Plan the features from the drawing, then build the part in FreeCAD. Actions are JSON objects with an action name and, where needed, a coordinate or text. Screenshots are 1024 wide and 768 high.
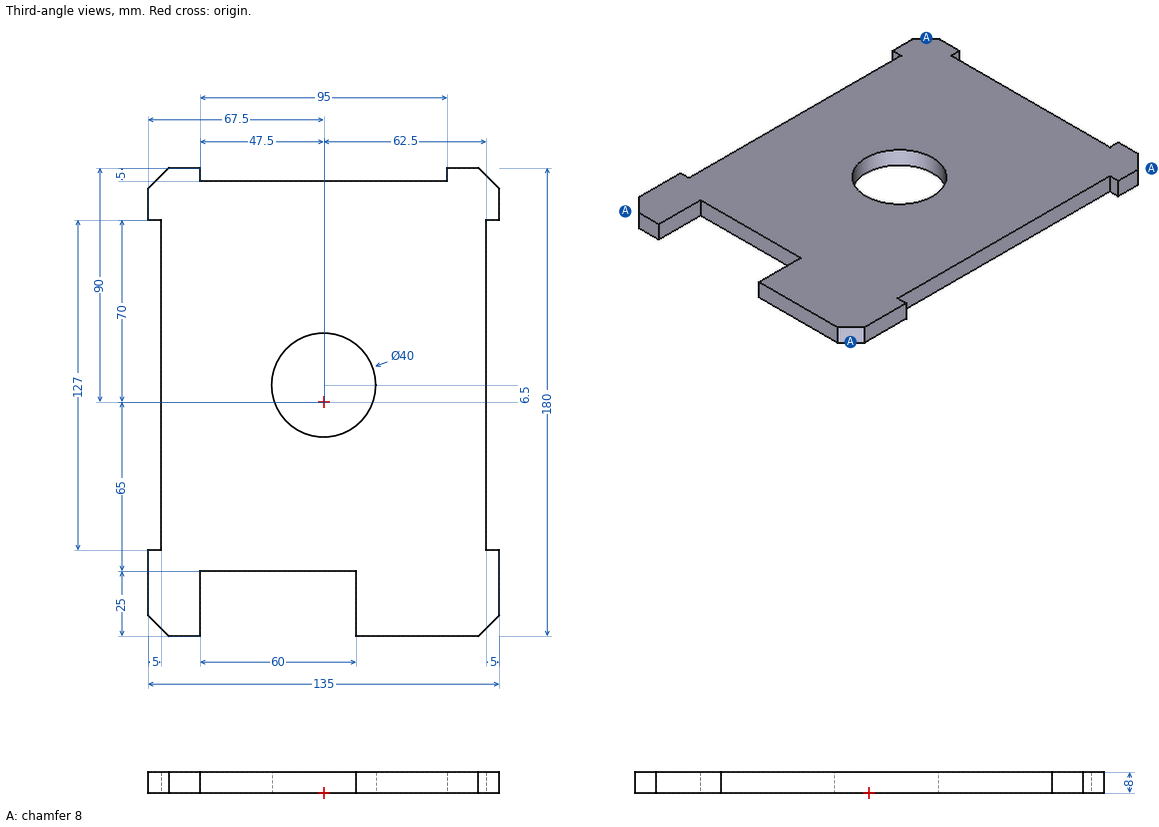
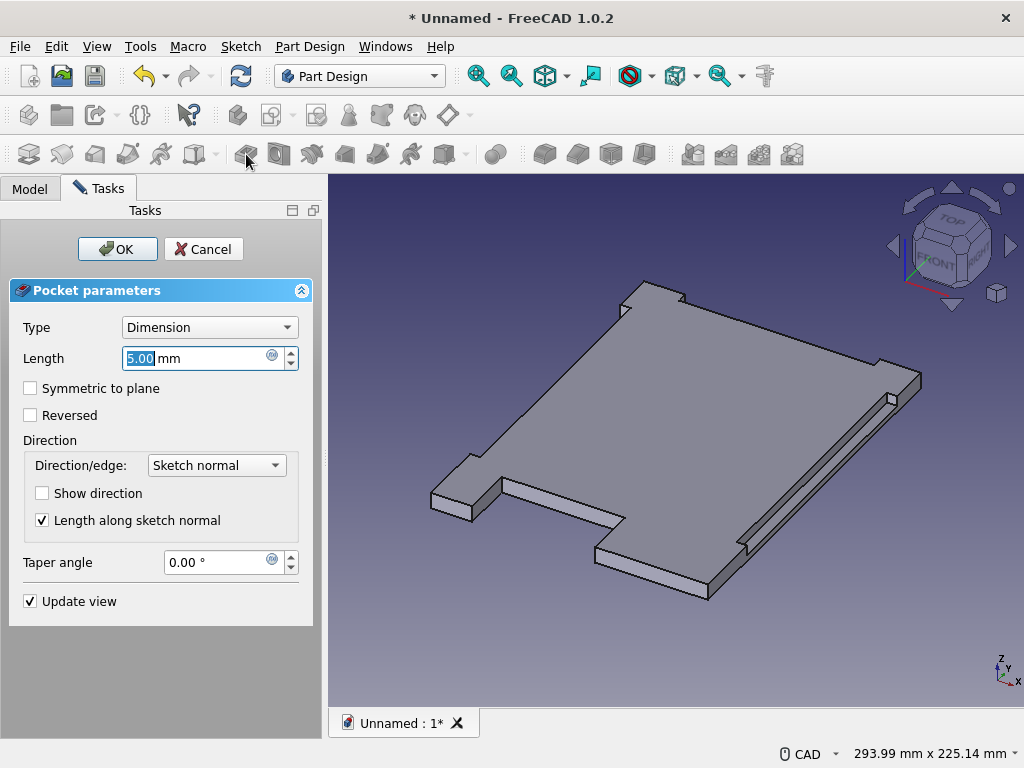
{"action": "left_click", "coordinate": [210, 328]}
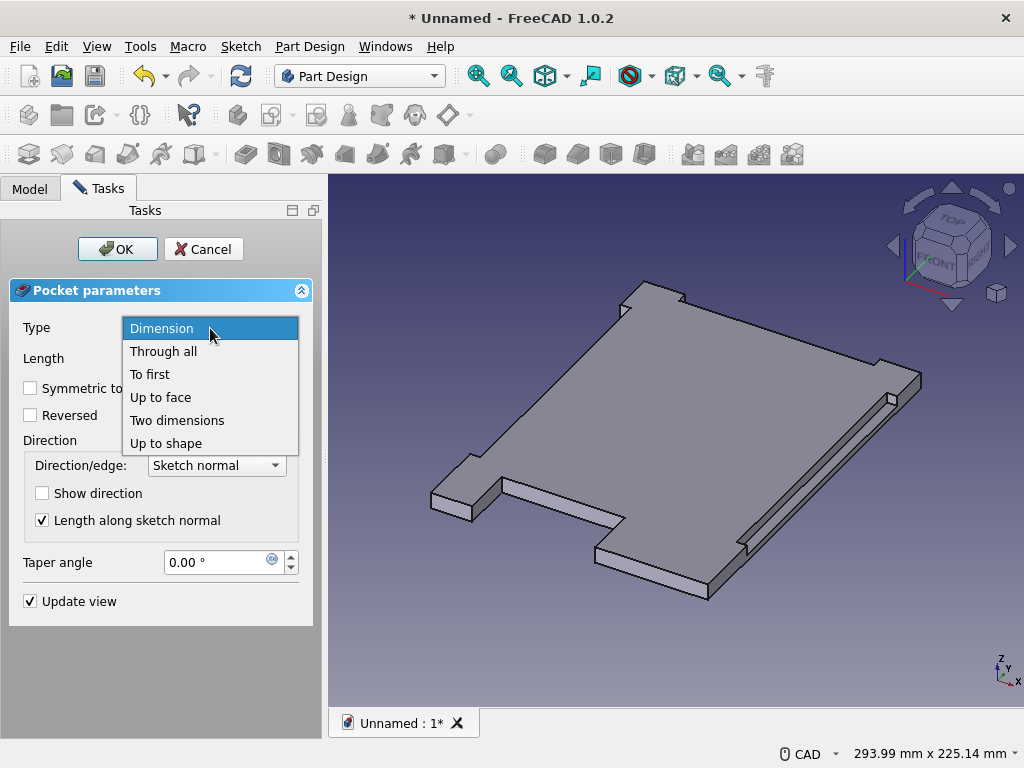
{"action": "left_click", "coordinate": [208, 374]}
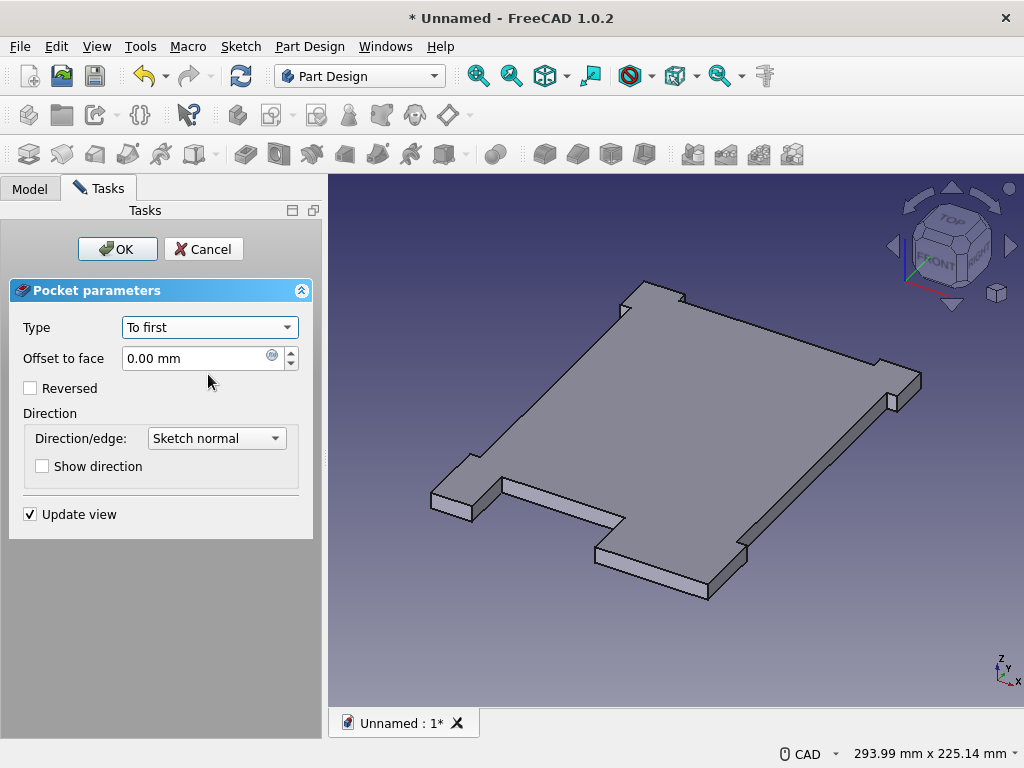
{"action": "left_click", "coordinate": [118, 249]}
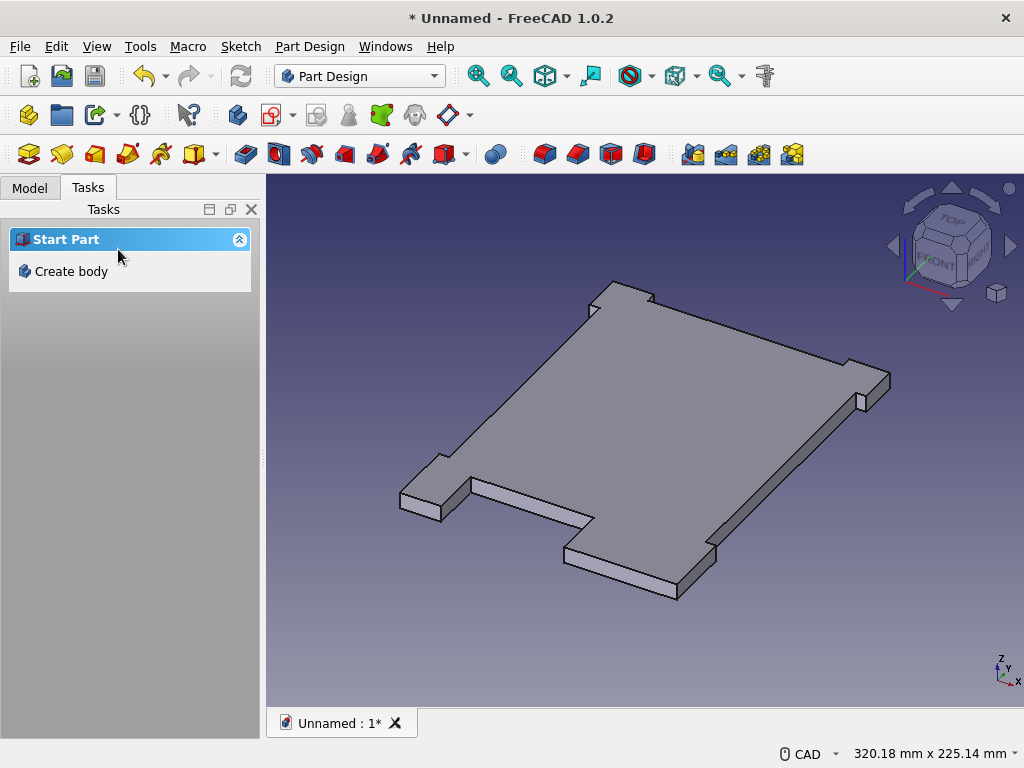
{"action": "left_click", "coordinate": [677, 591]}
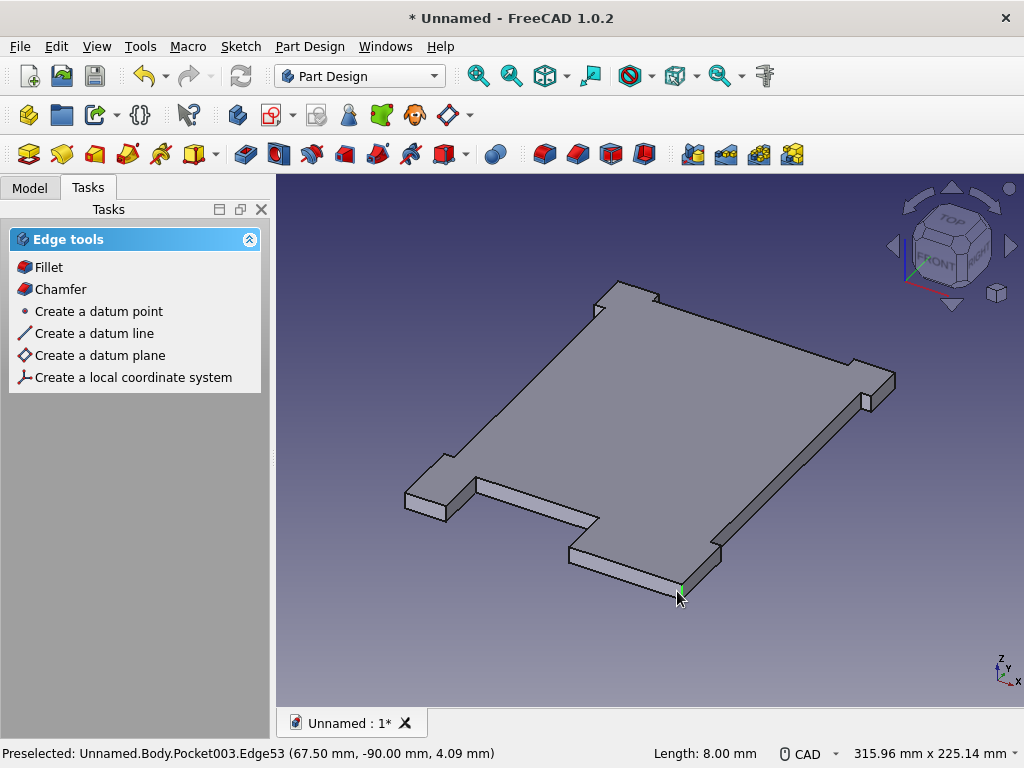
{"action": "scroll", "coordinate": [405, 500], "scroll_direction": "up", "scroll_amount": 4}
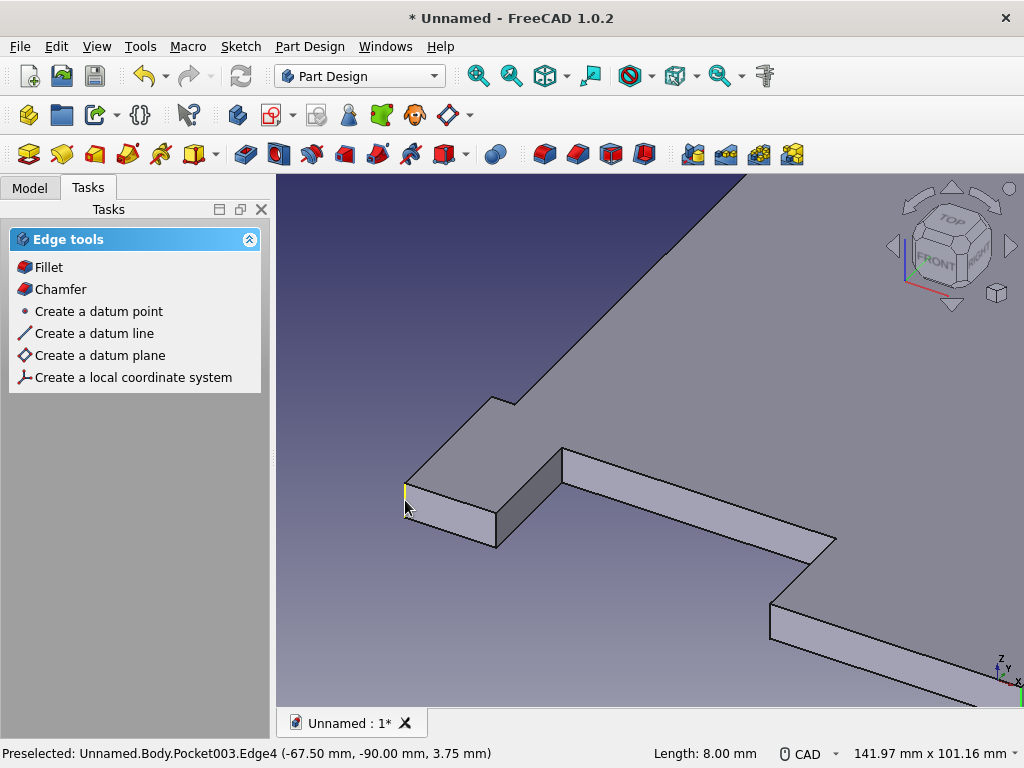
{"action": "key", "text": "v f"}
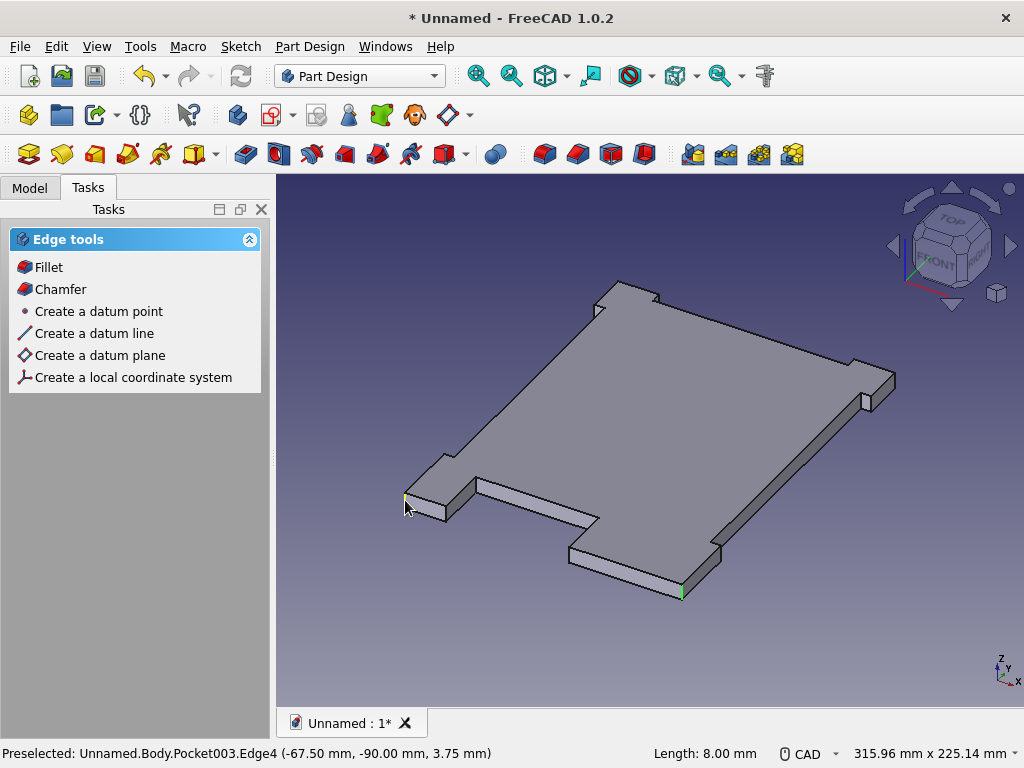
{"action": "key", "text": "0"}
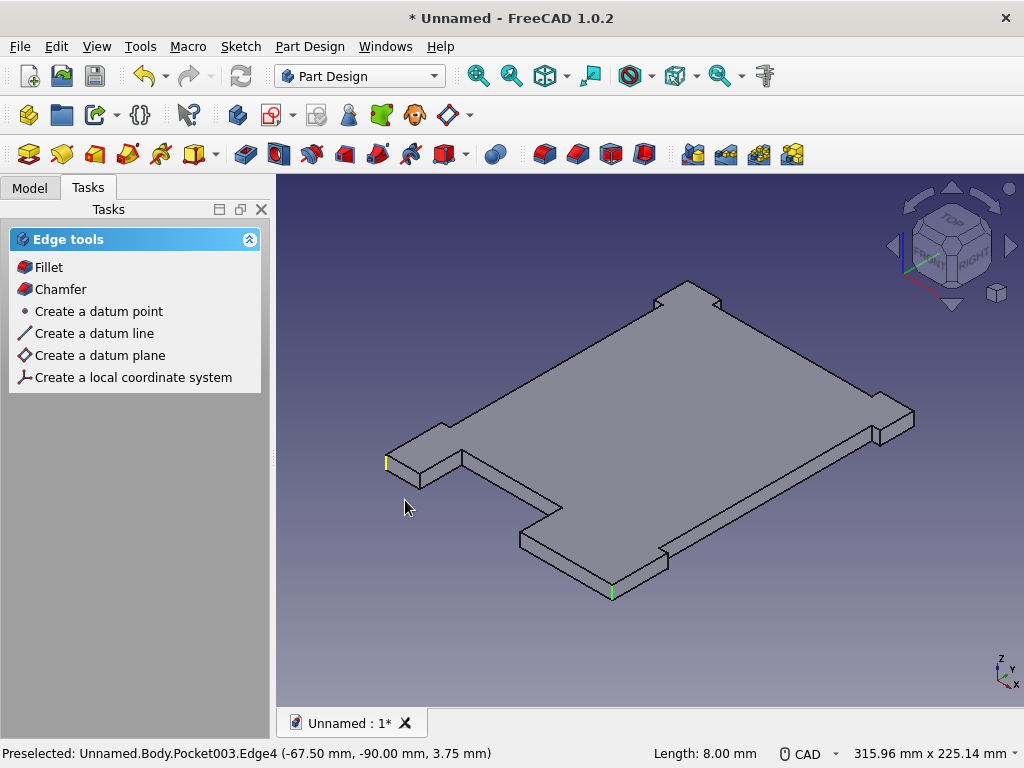
{"action": "scroll", "coordinate": [386, 461], "scroll_direction": "up", "scroll_amount": 4}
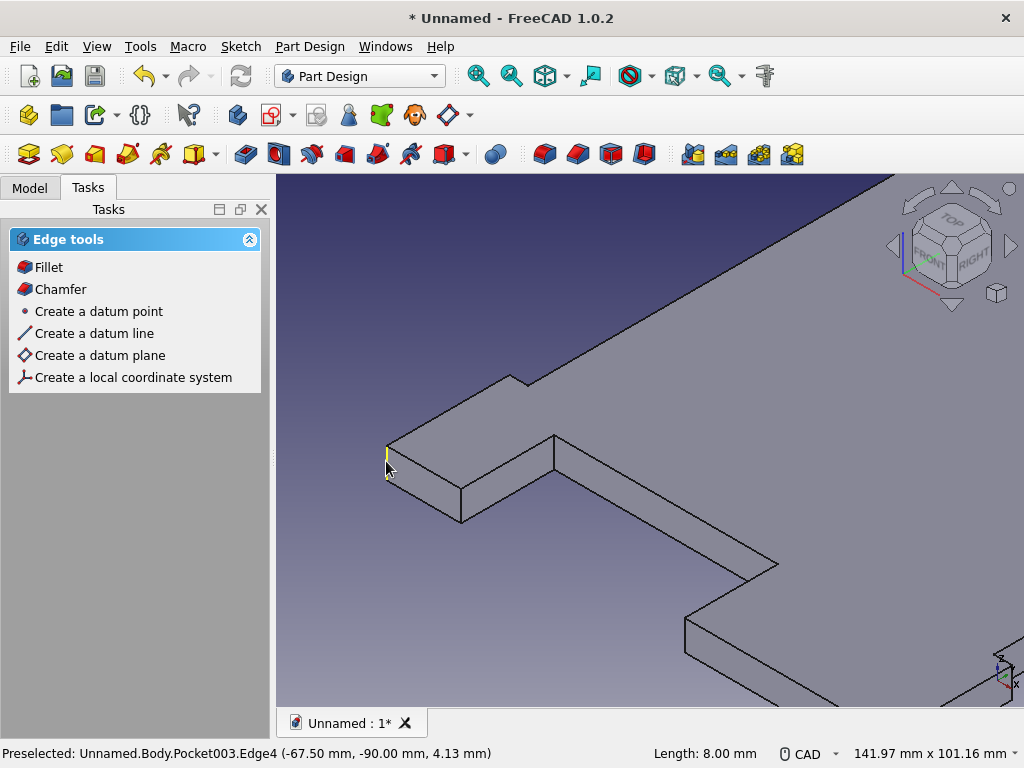
{"action": "left_click", "coordinate": [479, 76]}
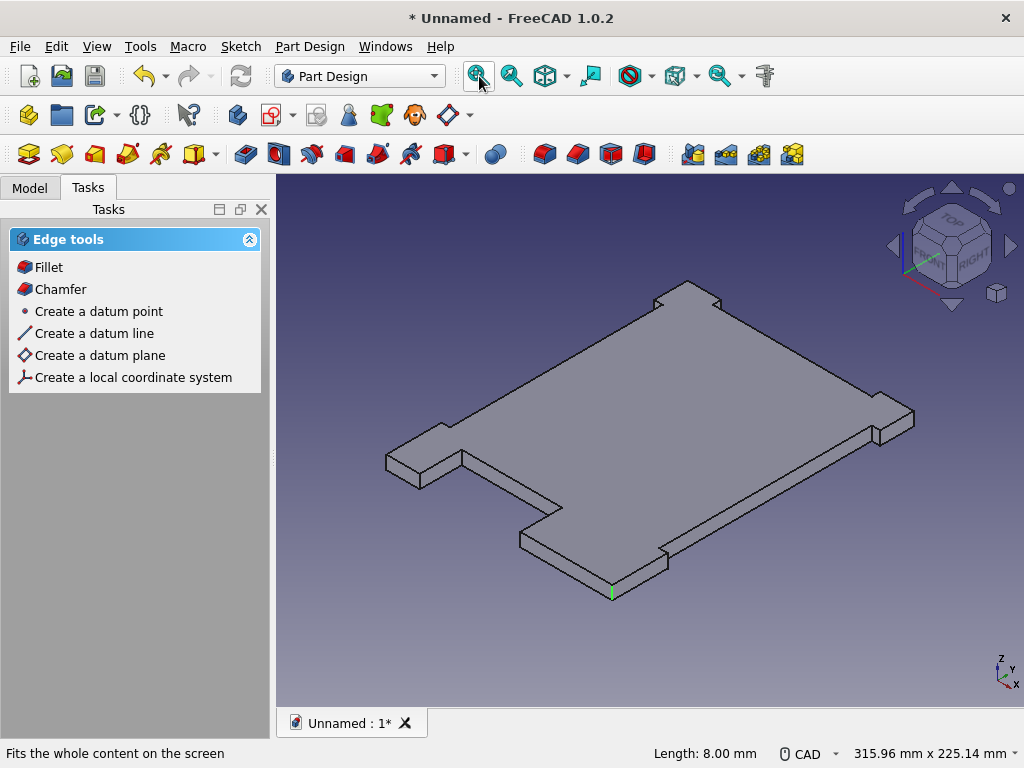
{"action": "key", "text": "2"}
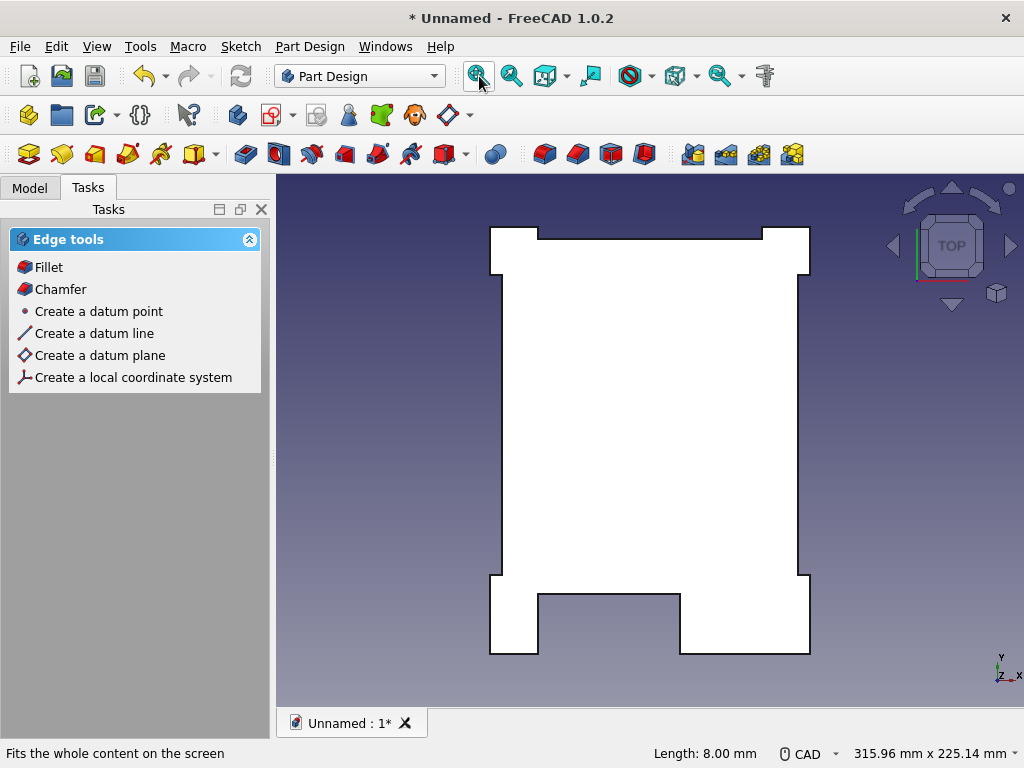
{"action": "scroll", "coordinate": [490, 653], "scroll_direction": "up", "scroll_amount": 4}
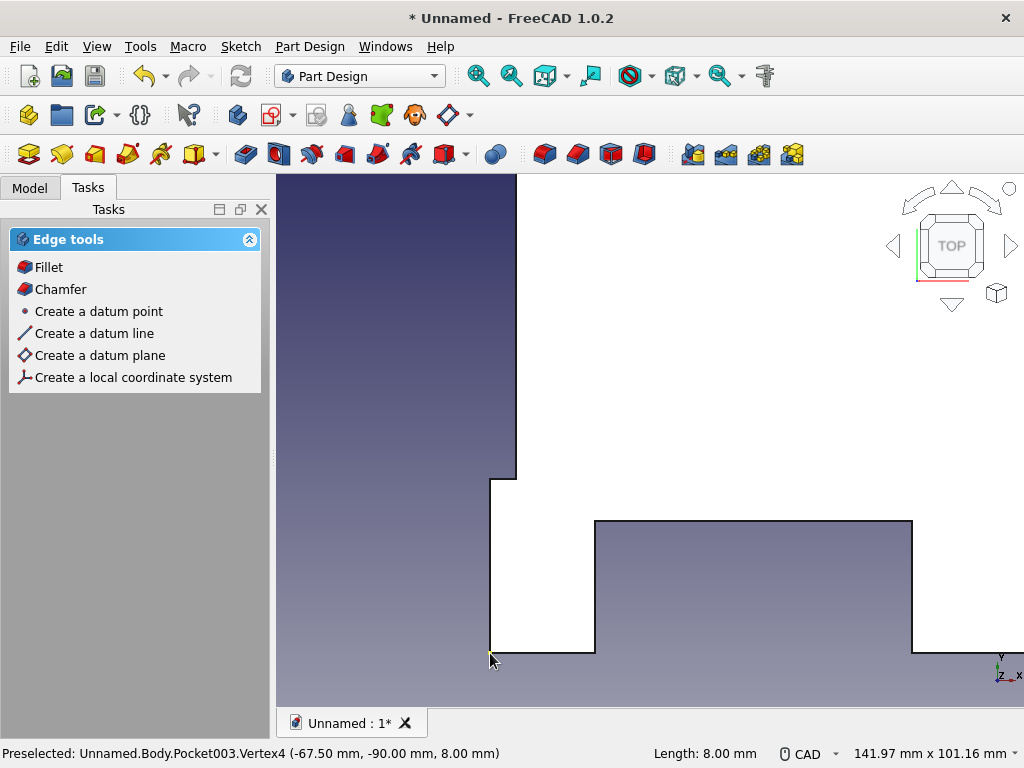
{"action": "key", "text": "v f"}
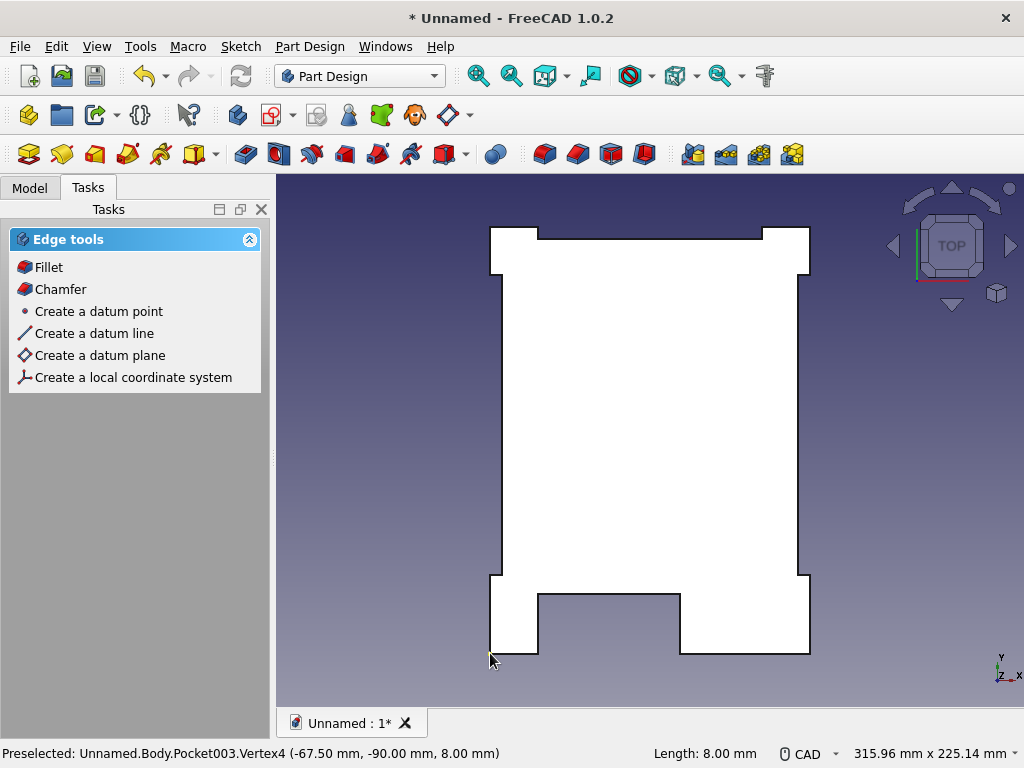
{"action": "key", "text": "1"}